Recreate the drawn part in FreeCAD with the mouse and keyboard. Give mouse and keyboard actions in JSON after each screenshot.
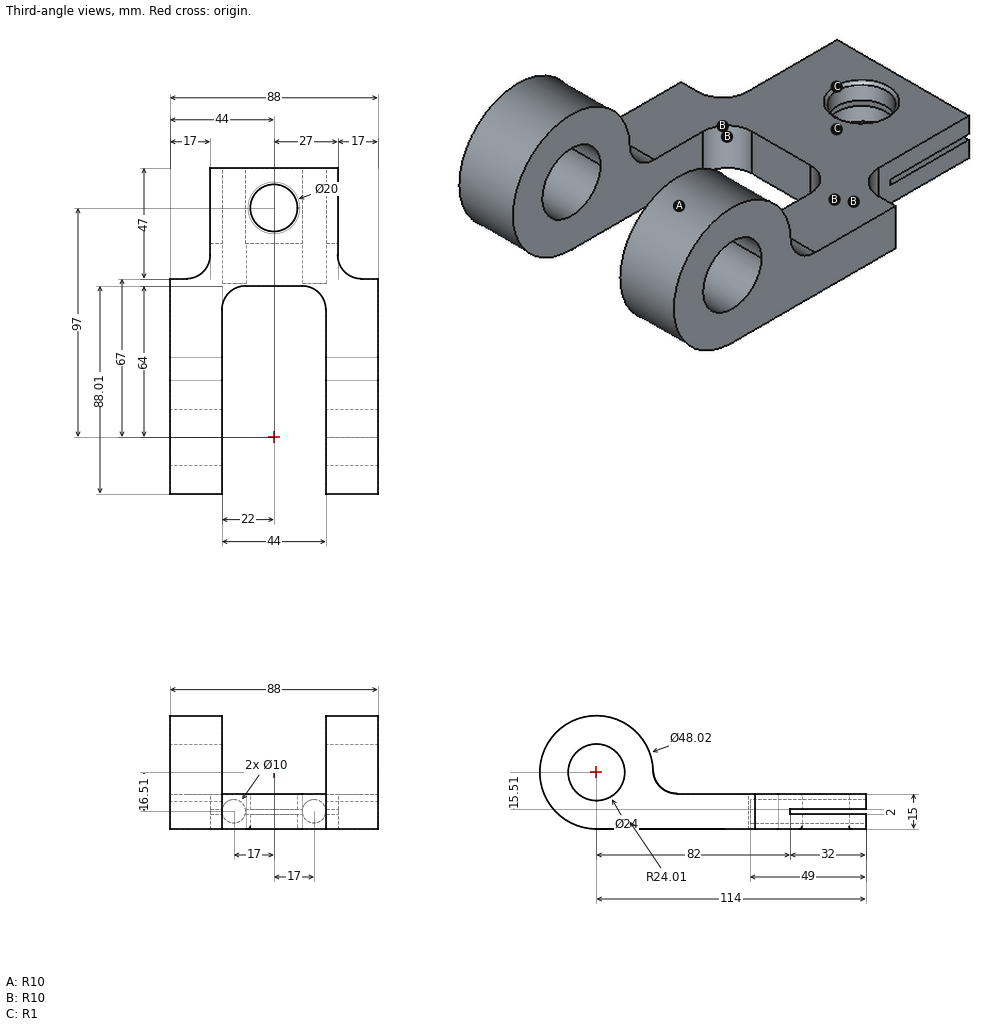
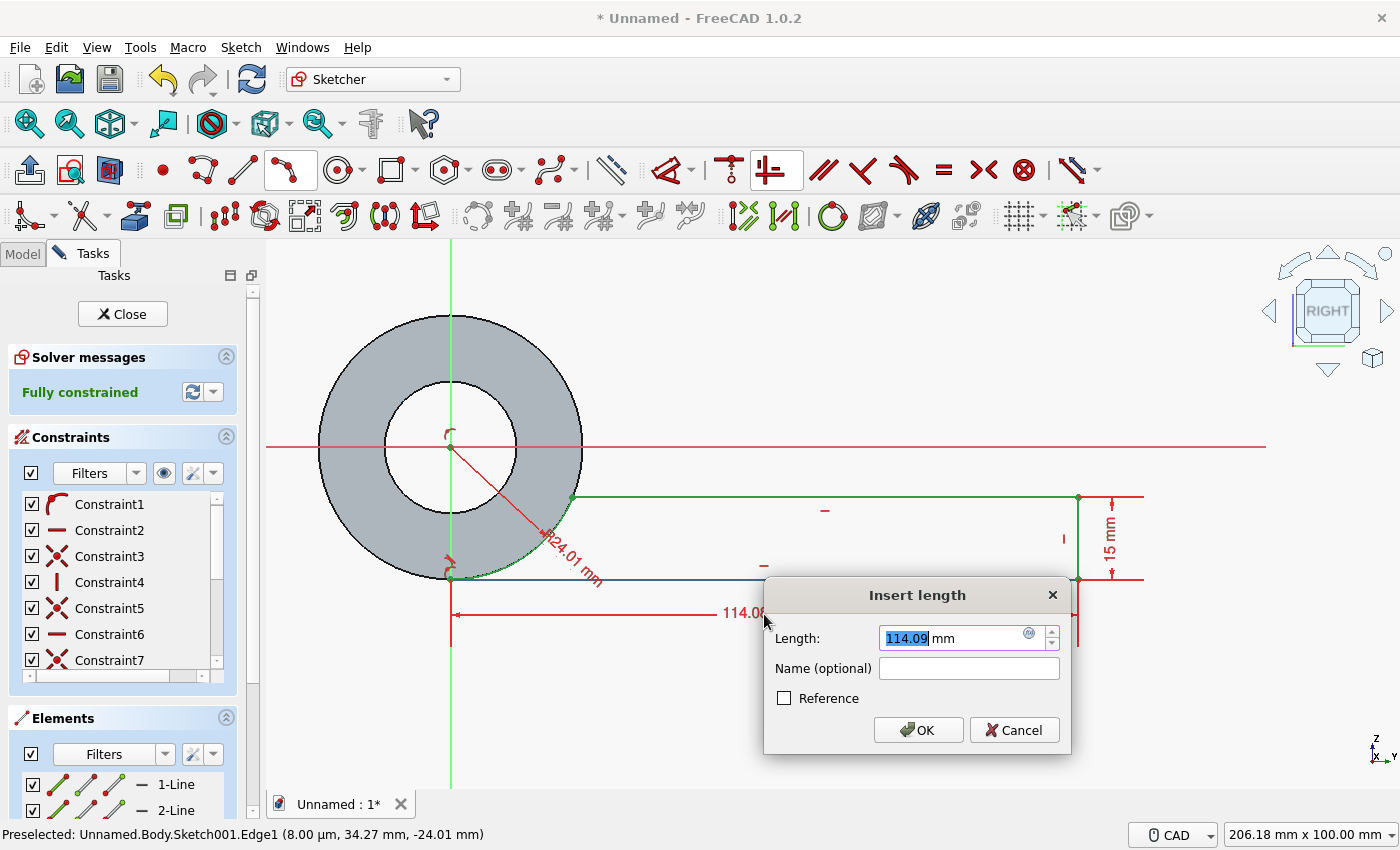
{"action": "type", "text": "114"}
{"action": "key", "text": "Return"}
{"action": "key", "text": "Escape"}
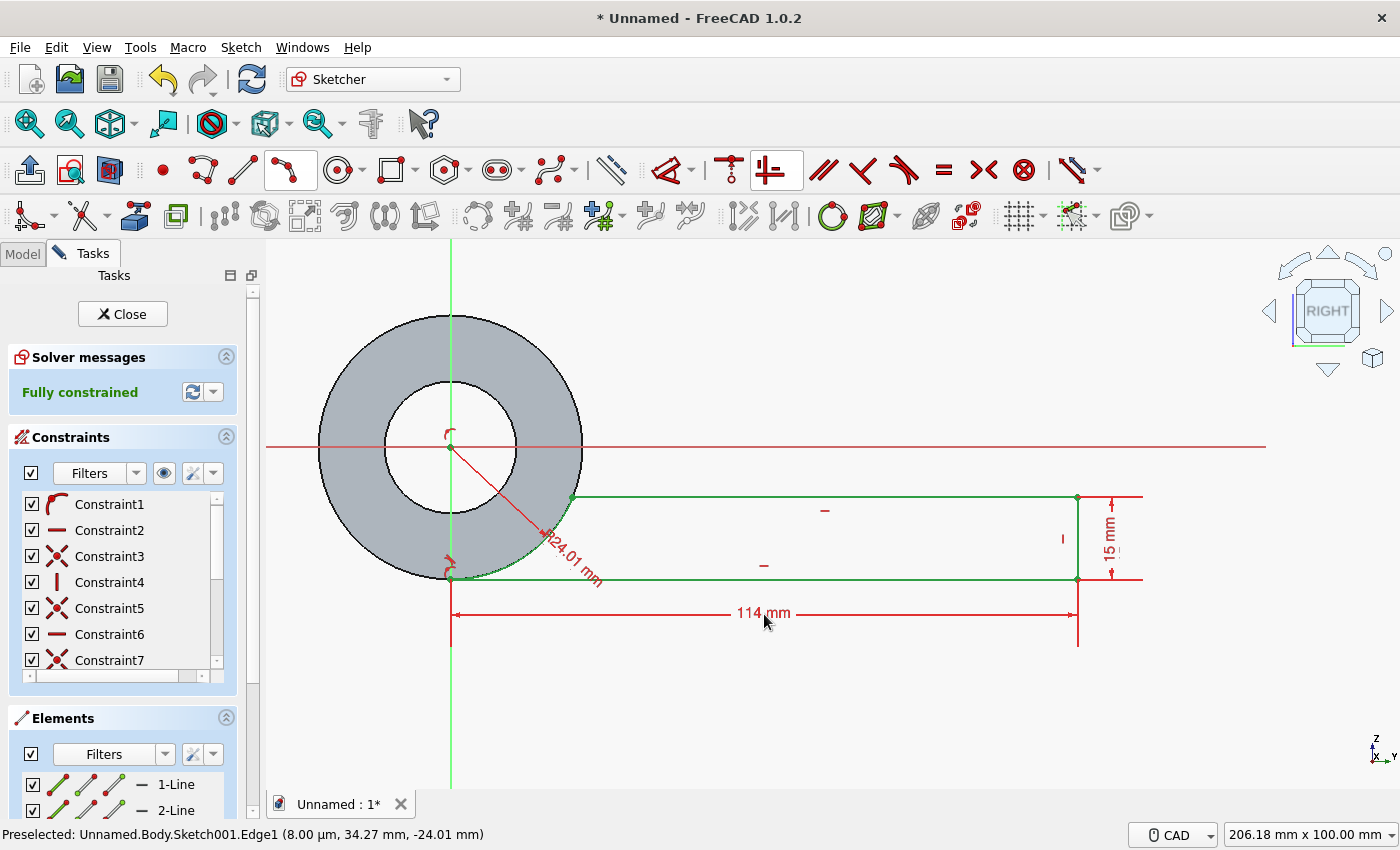
{"action": "left_click", "coordinate": [123, 314]}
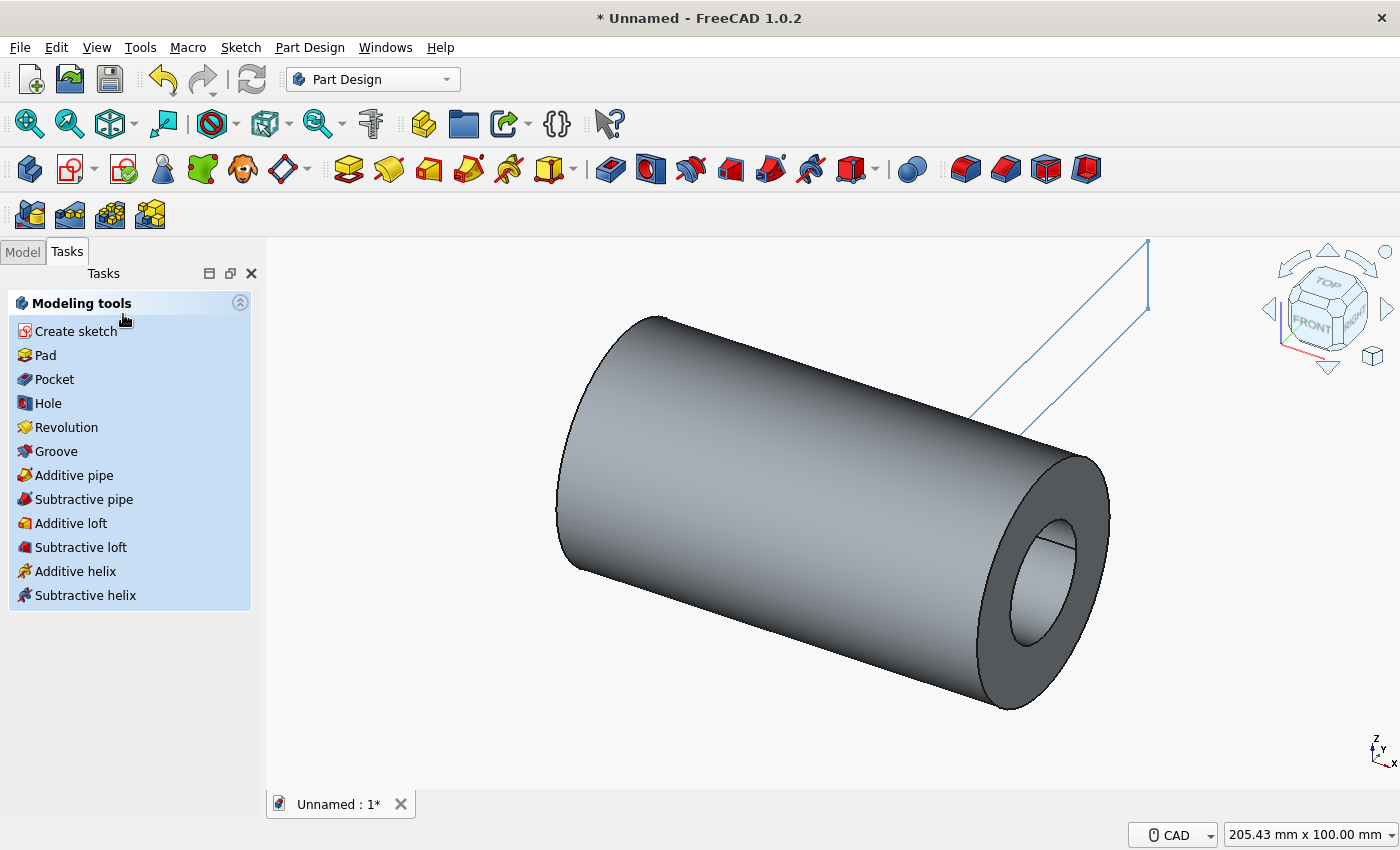
{"action": "left_click", "coordinate": [350, 170]}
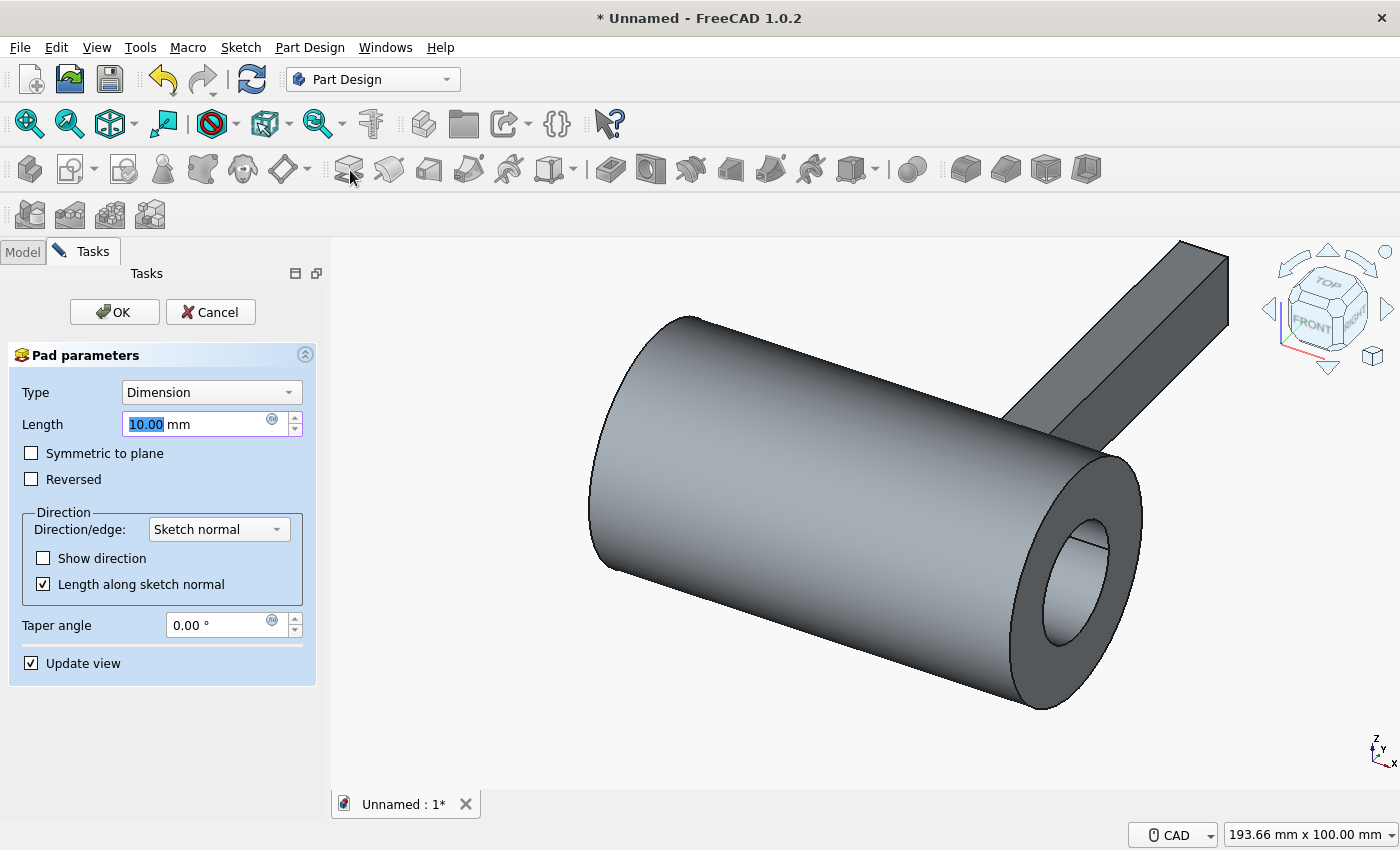
{"action": "type", "text": "88"}
{"action": "key", "text": "Tab"}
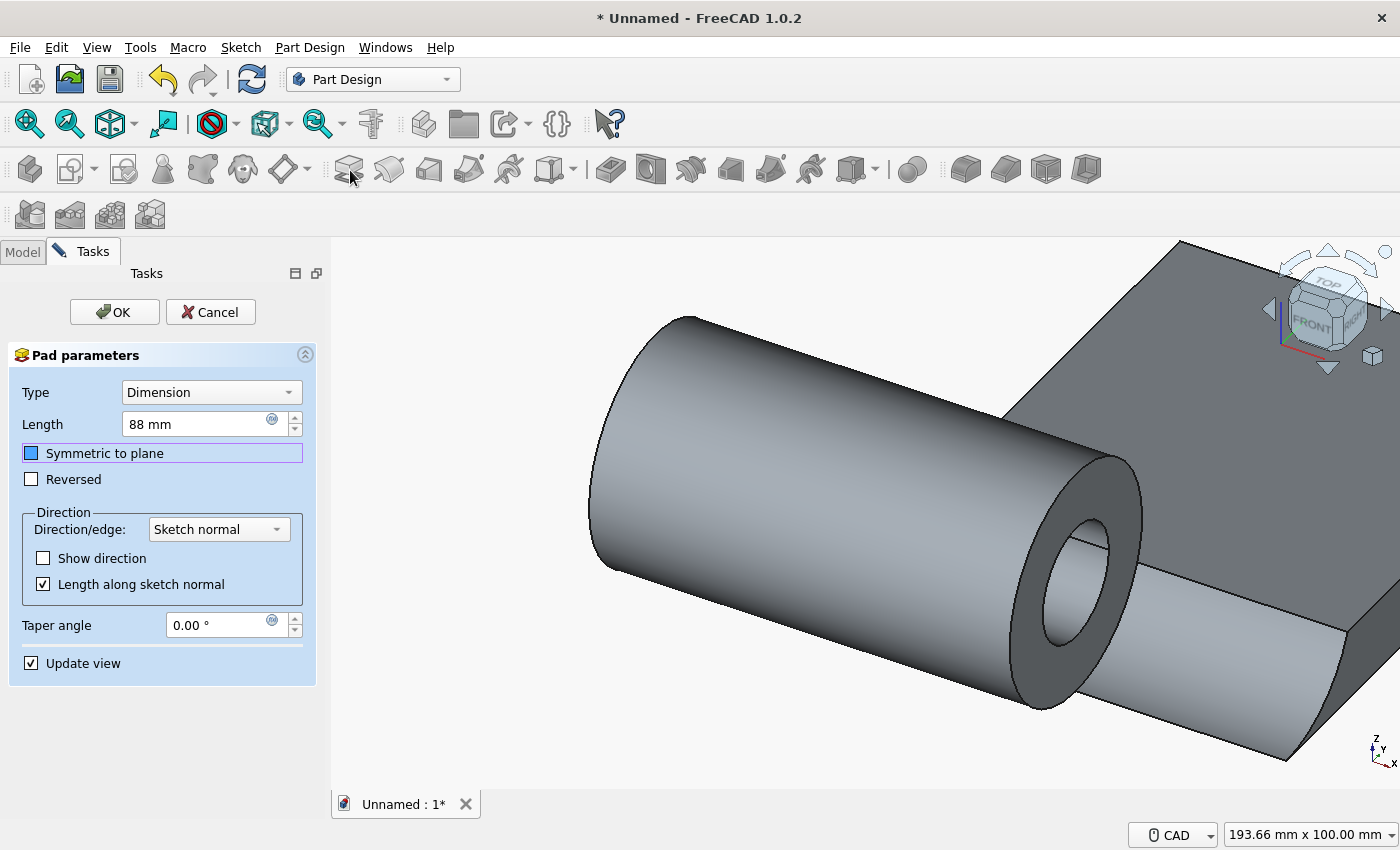
{"action": "left_click", "coordinate": [30, 453]}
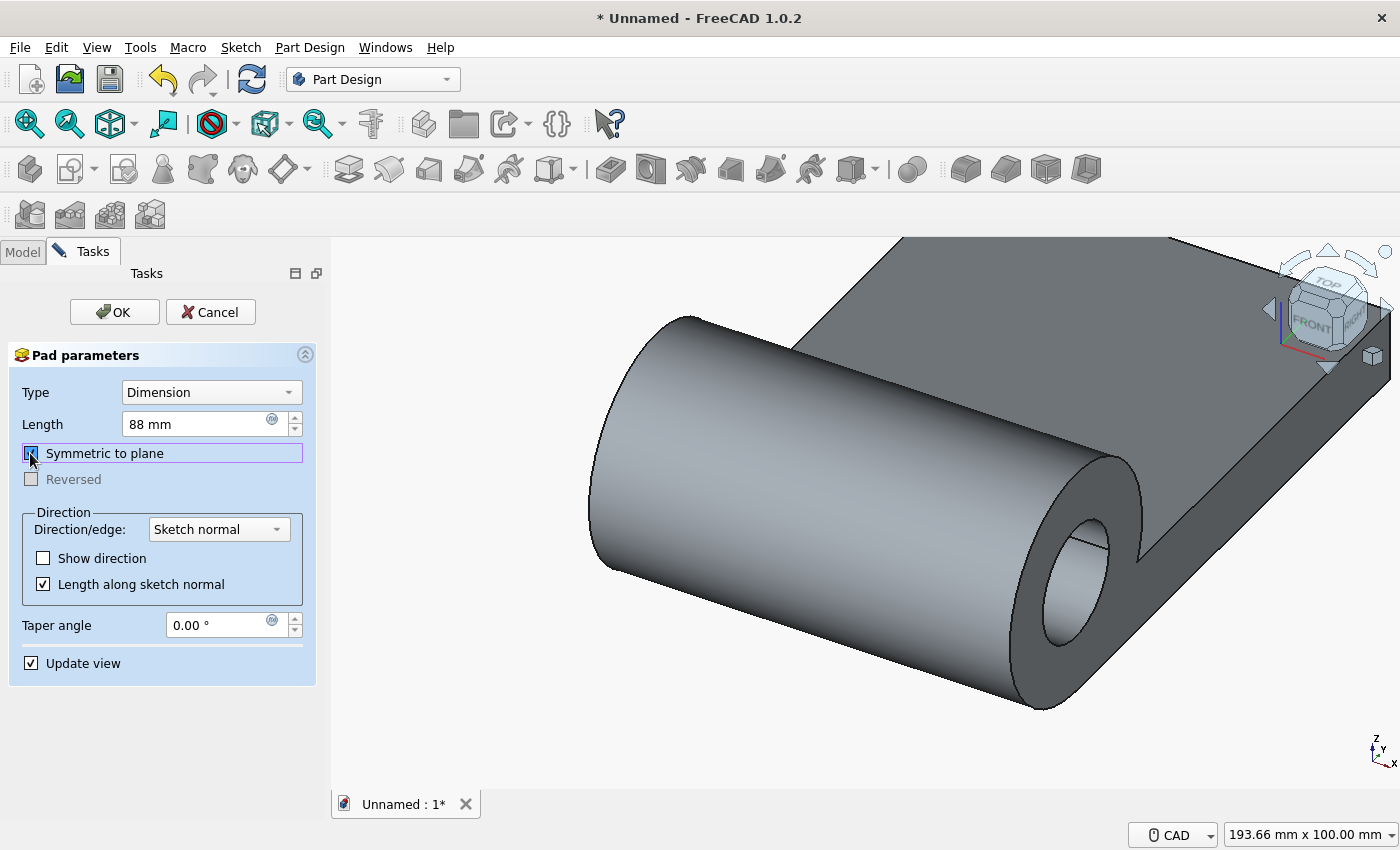
{"action": "left_click", "coordinate": [115, 312]}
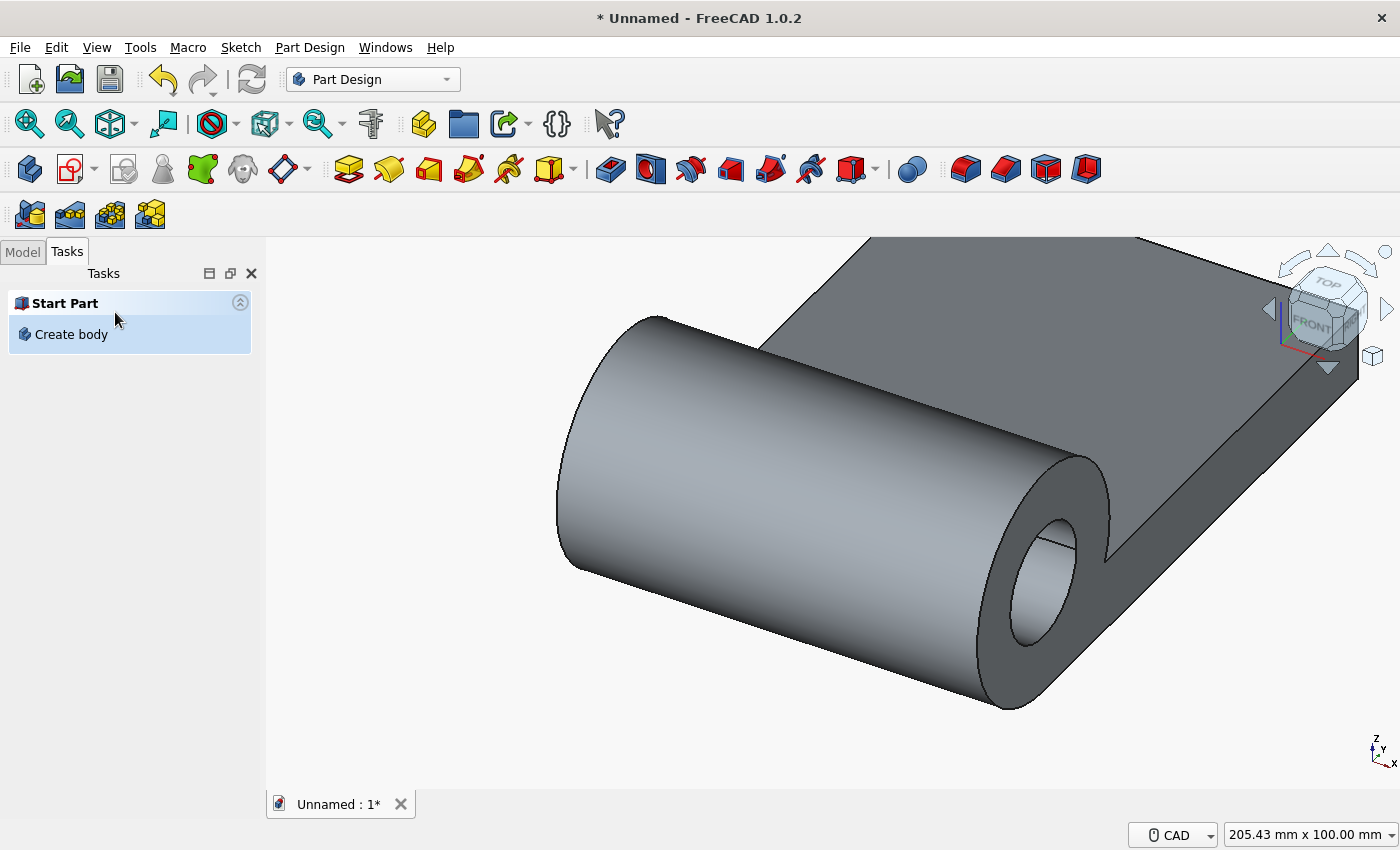
{"action": "left_click", "coordinate": [30, 124]}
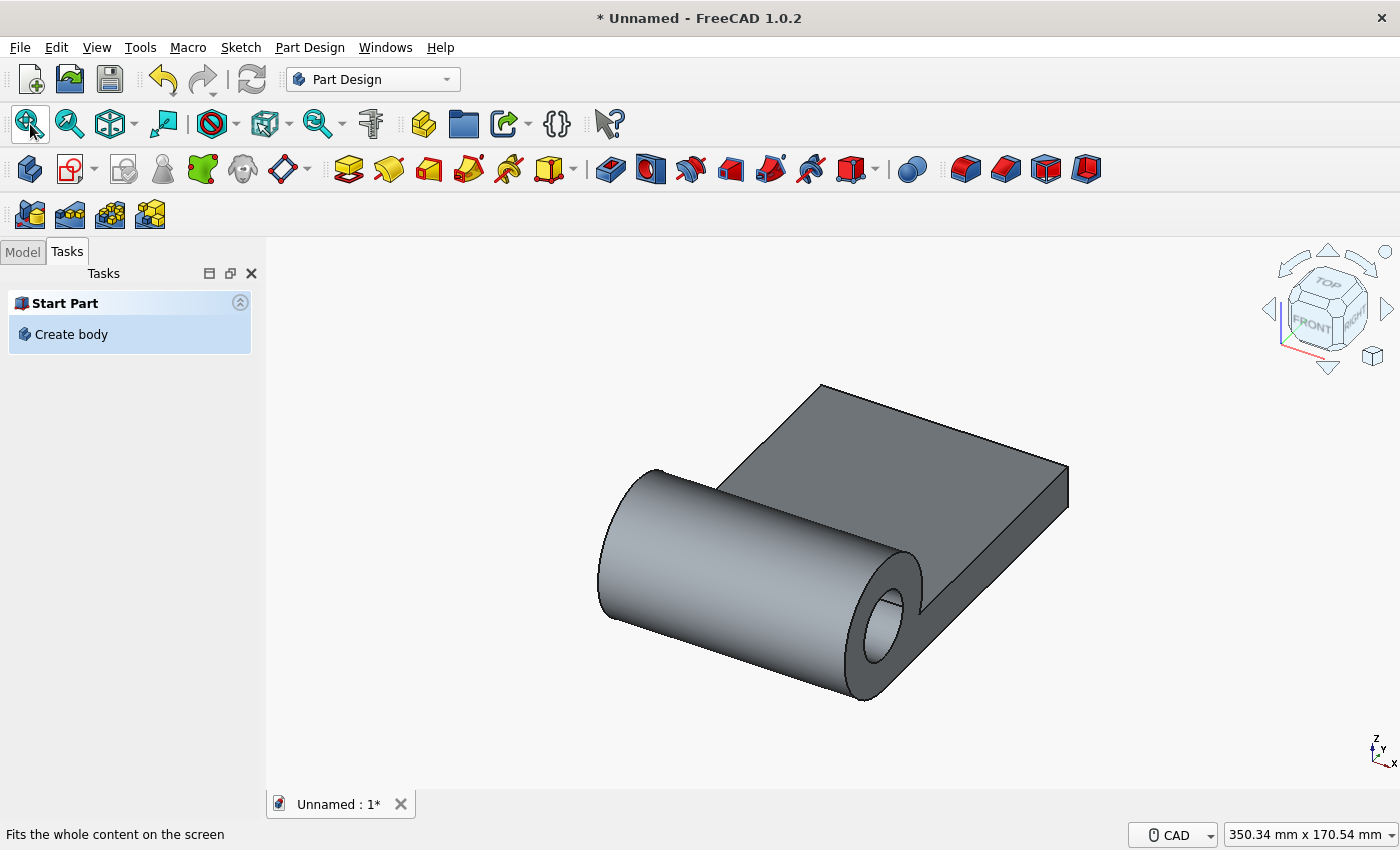
{"action": "key", "text": "0"}